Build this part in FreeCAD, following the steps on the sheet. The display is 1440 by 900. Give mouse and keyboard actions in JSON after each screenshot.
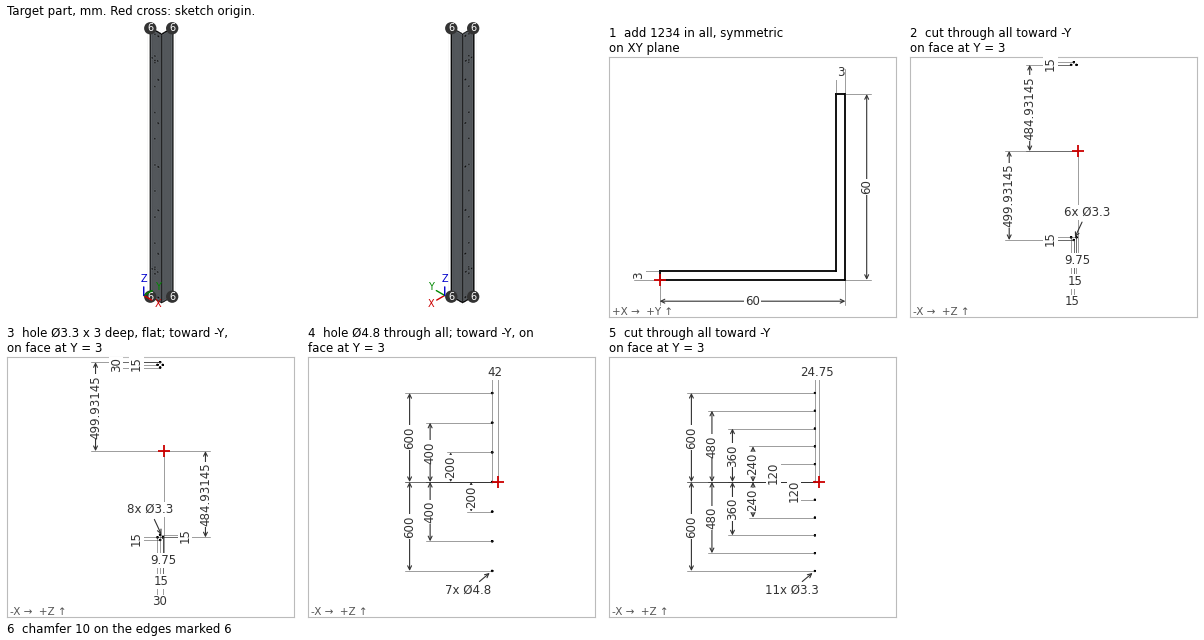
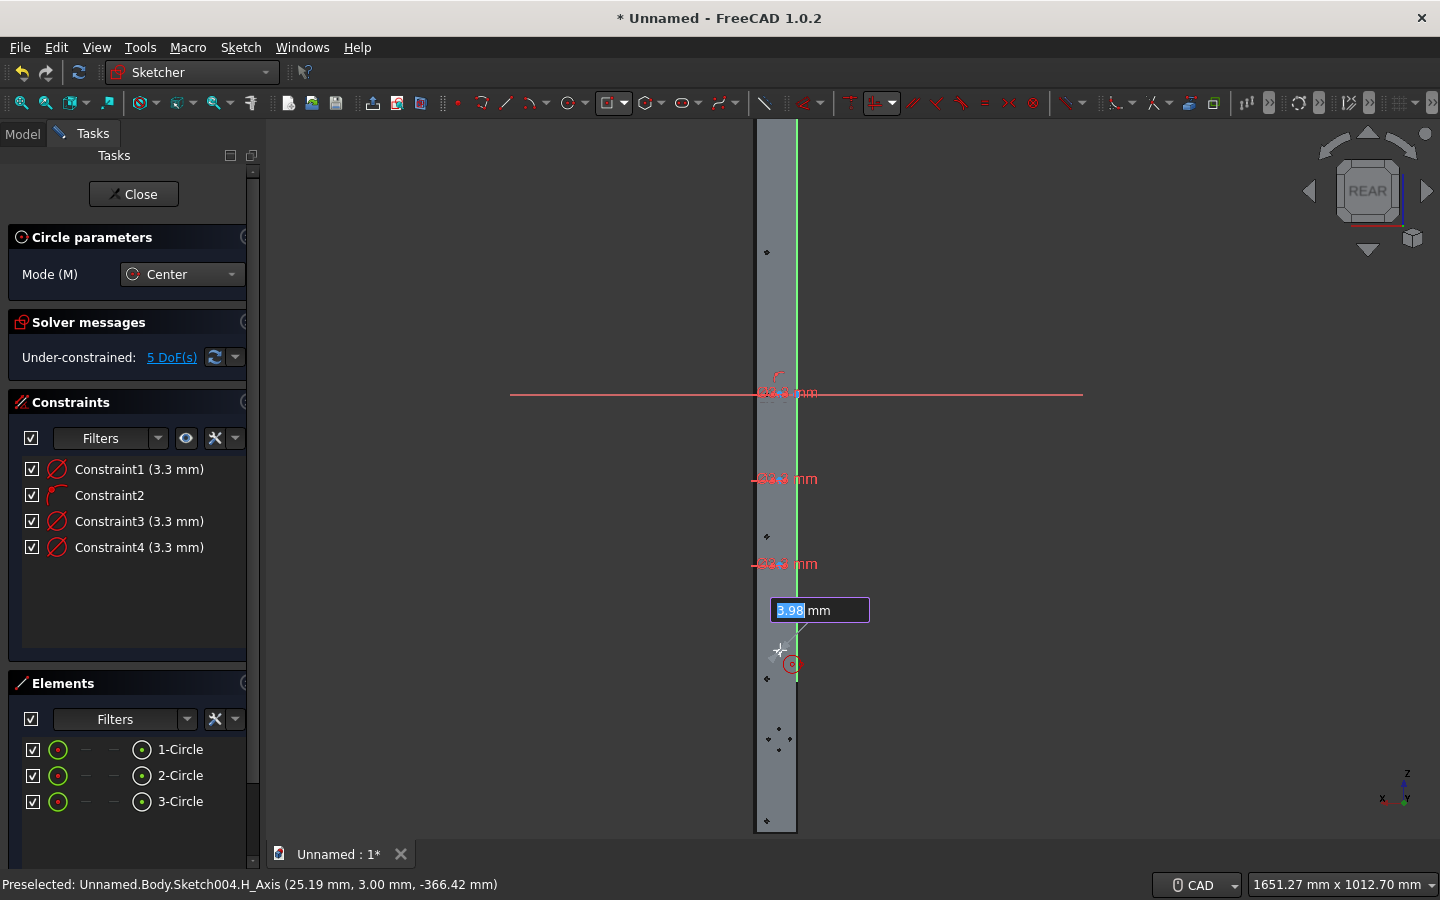
{"action": "type", "text": "3.3"}
{"action": "key", "text": "Return"}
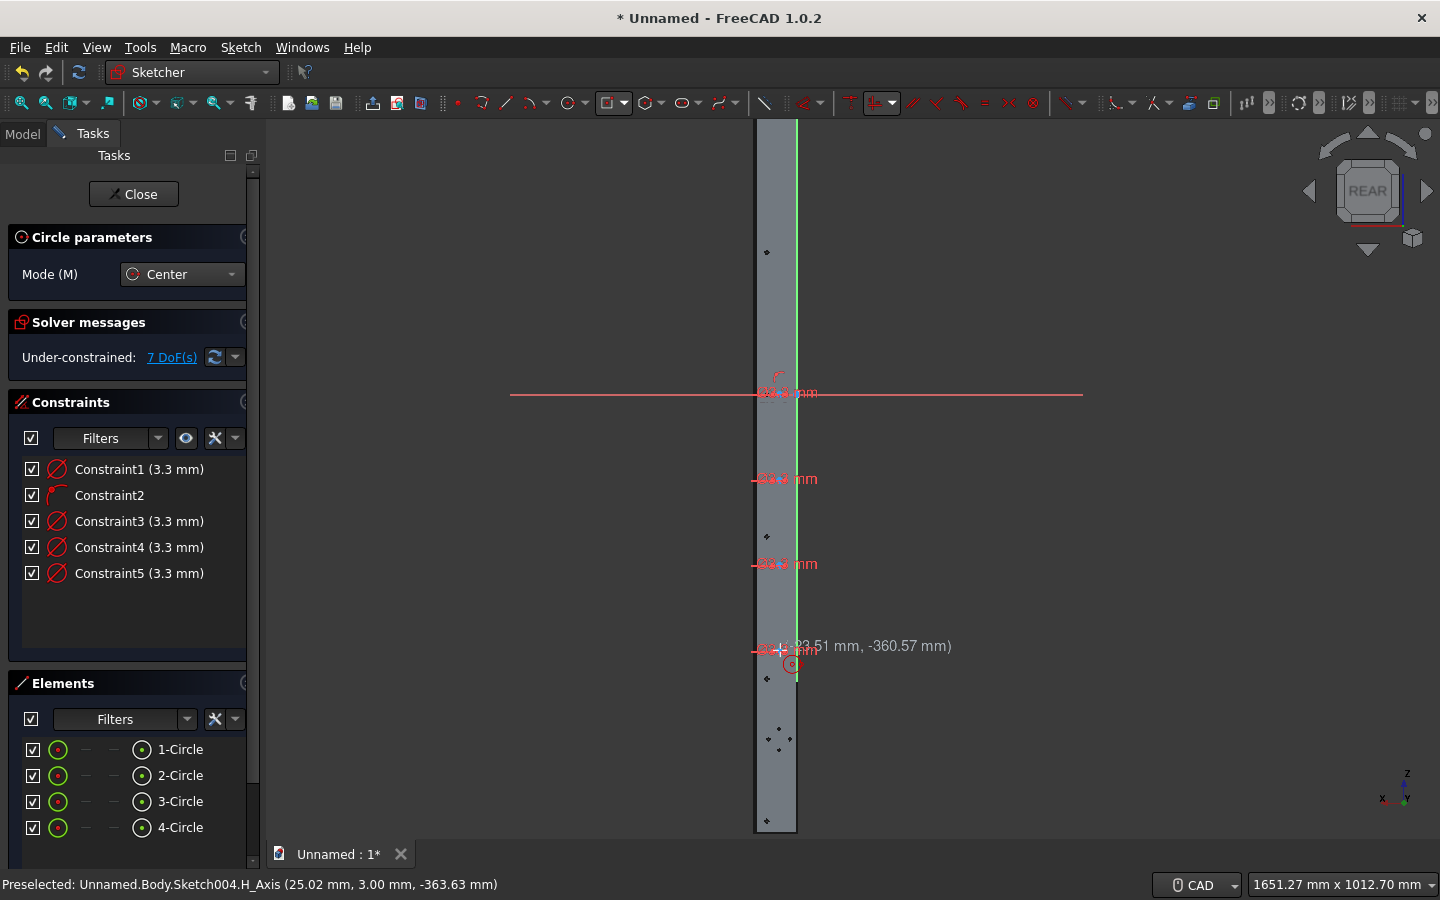
{"action": "scroll", "coordinate": [779, 736], "scroll_direction": "up", "scroll_amount": 15}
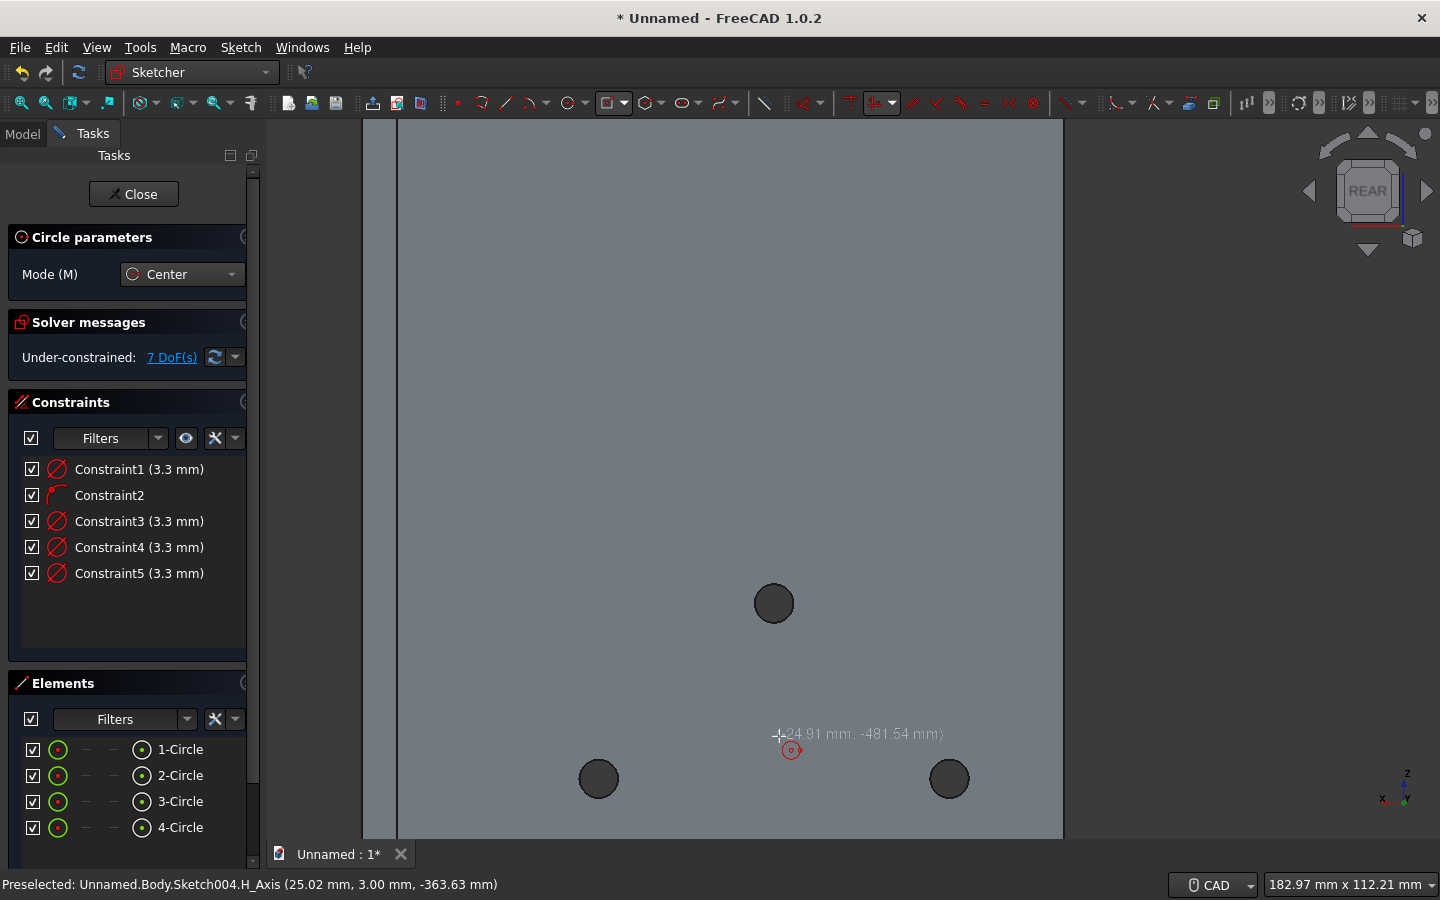
{"action": "scroll", "coordinate": [779, 707], "scroll_direction": "down", "scroll_amount": 17}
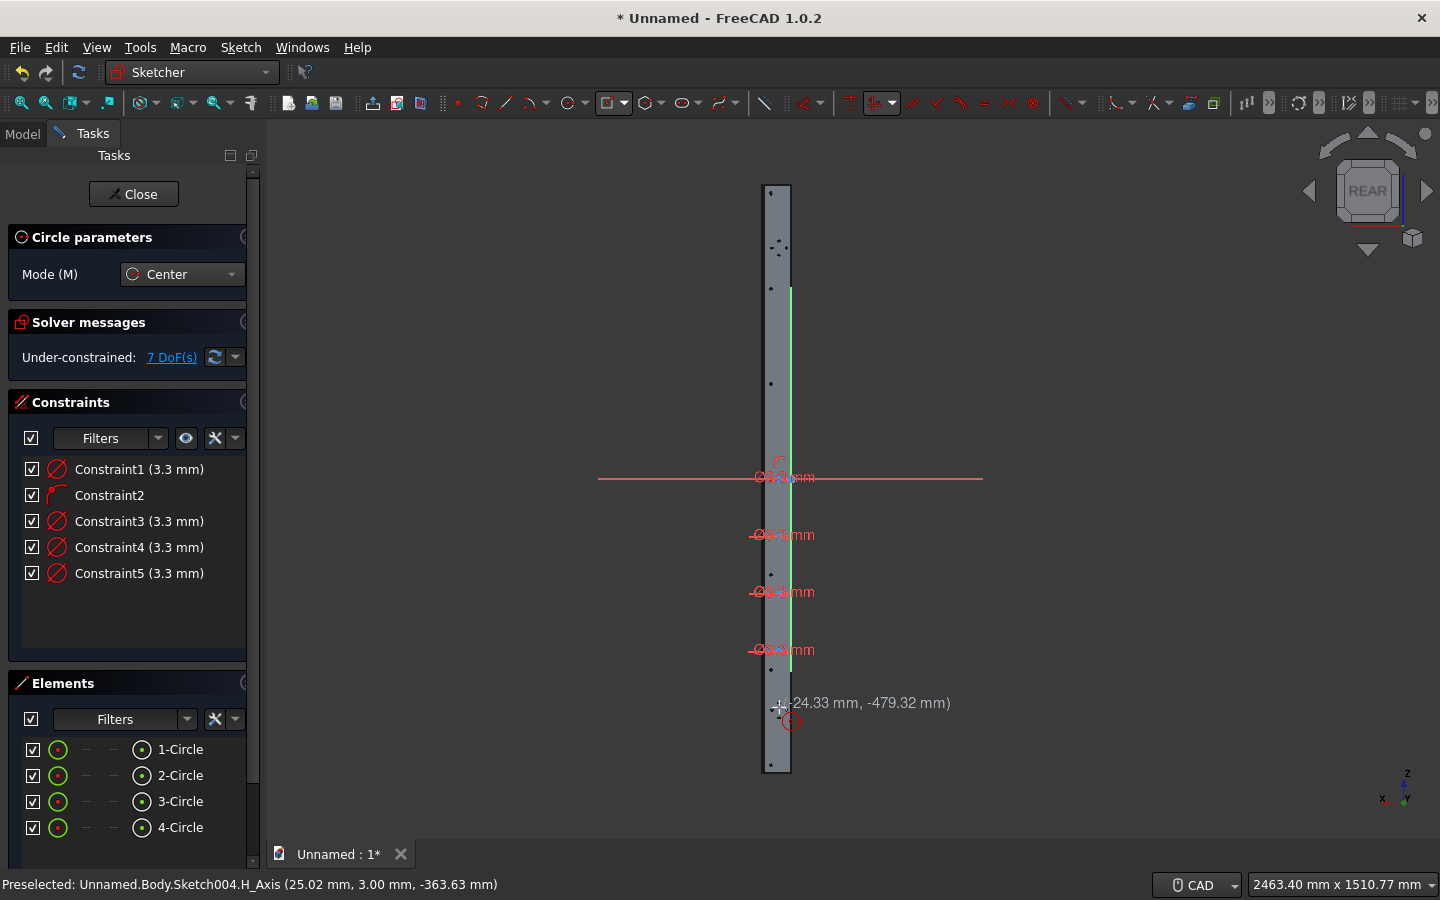
{"action": "scroll", "coordinate": [779, 708], "scroll_direction": "up", "scroll_amount": 2}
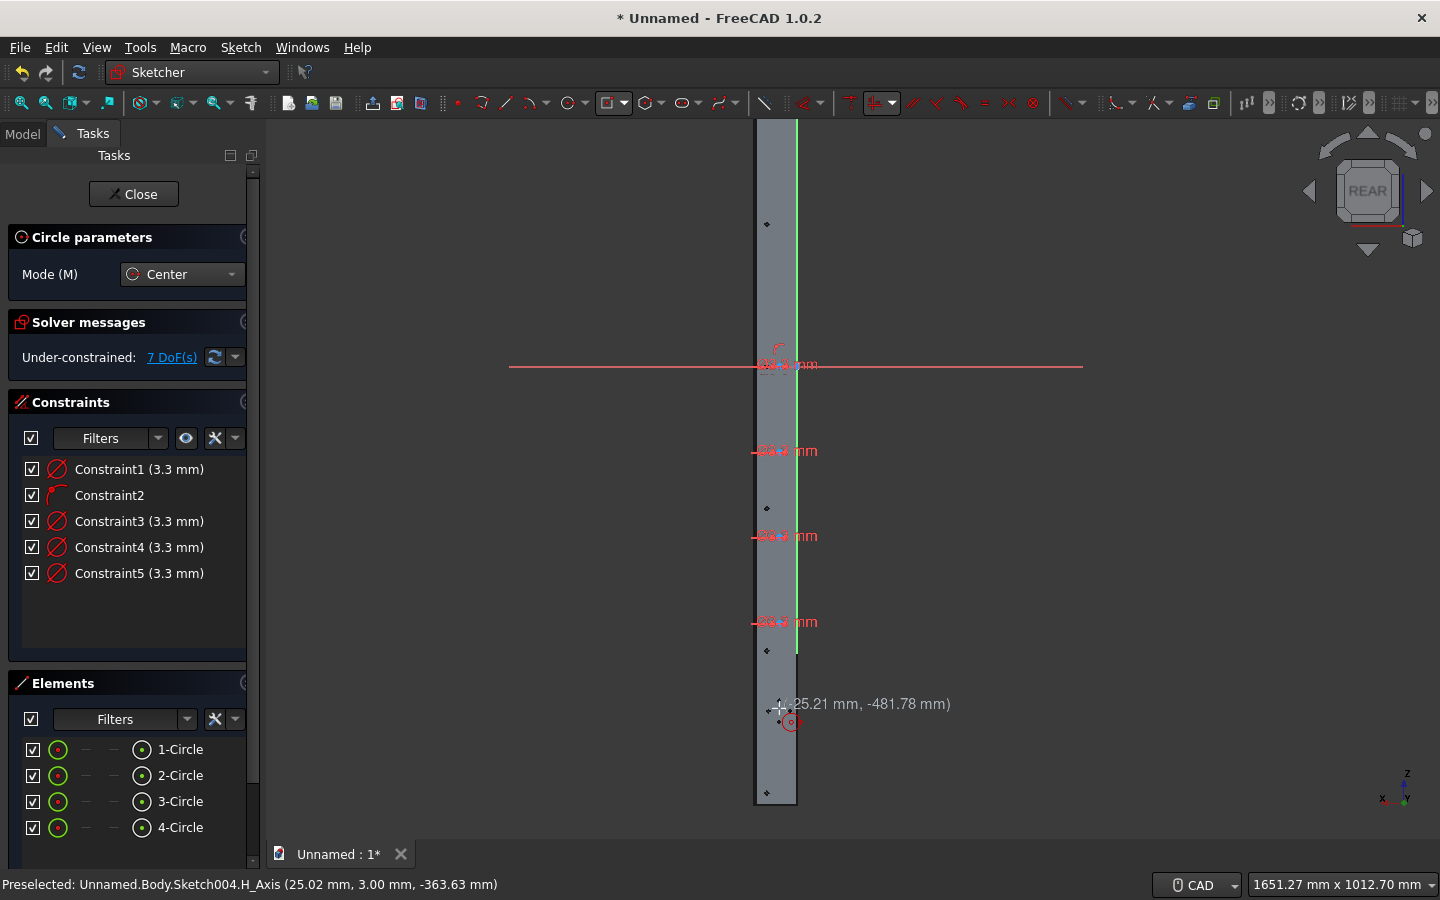
{"action": "left_click", "coordinate": [779, 708]}
{"action": "mouse_move", "coordinate": [780, 707]}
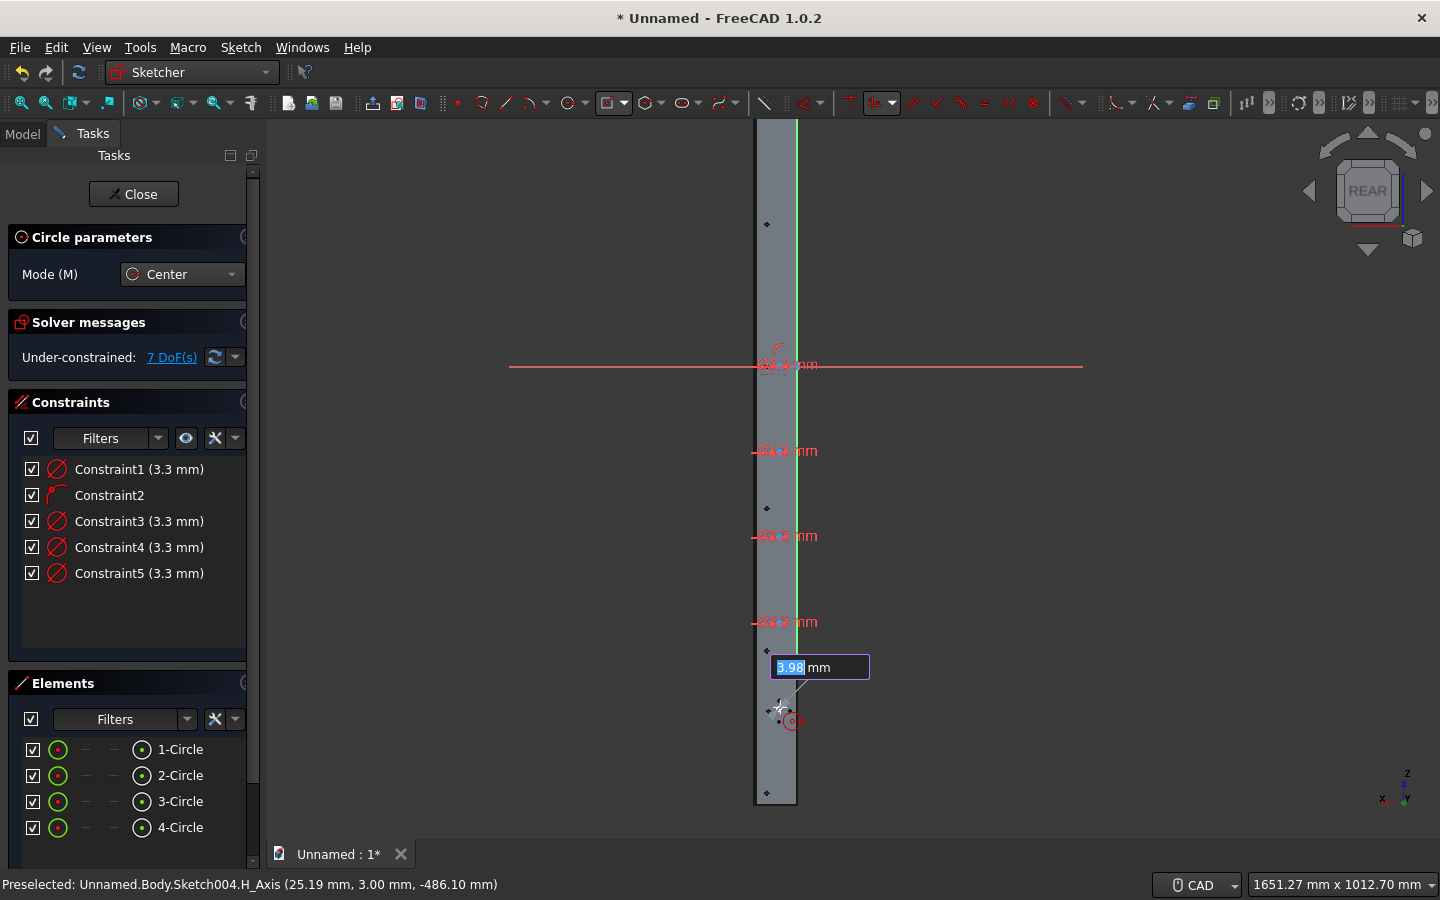
{"action": "type", "text": "3.3"}
{"action": "key", "text": "Return"}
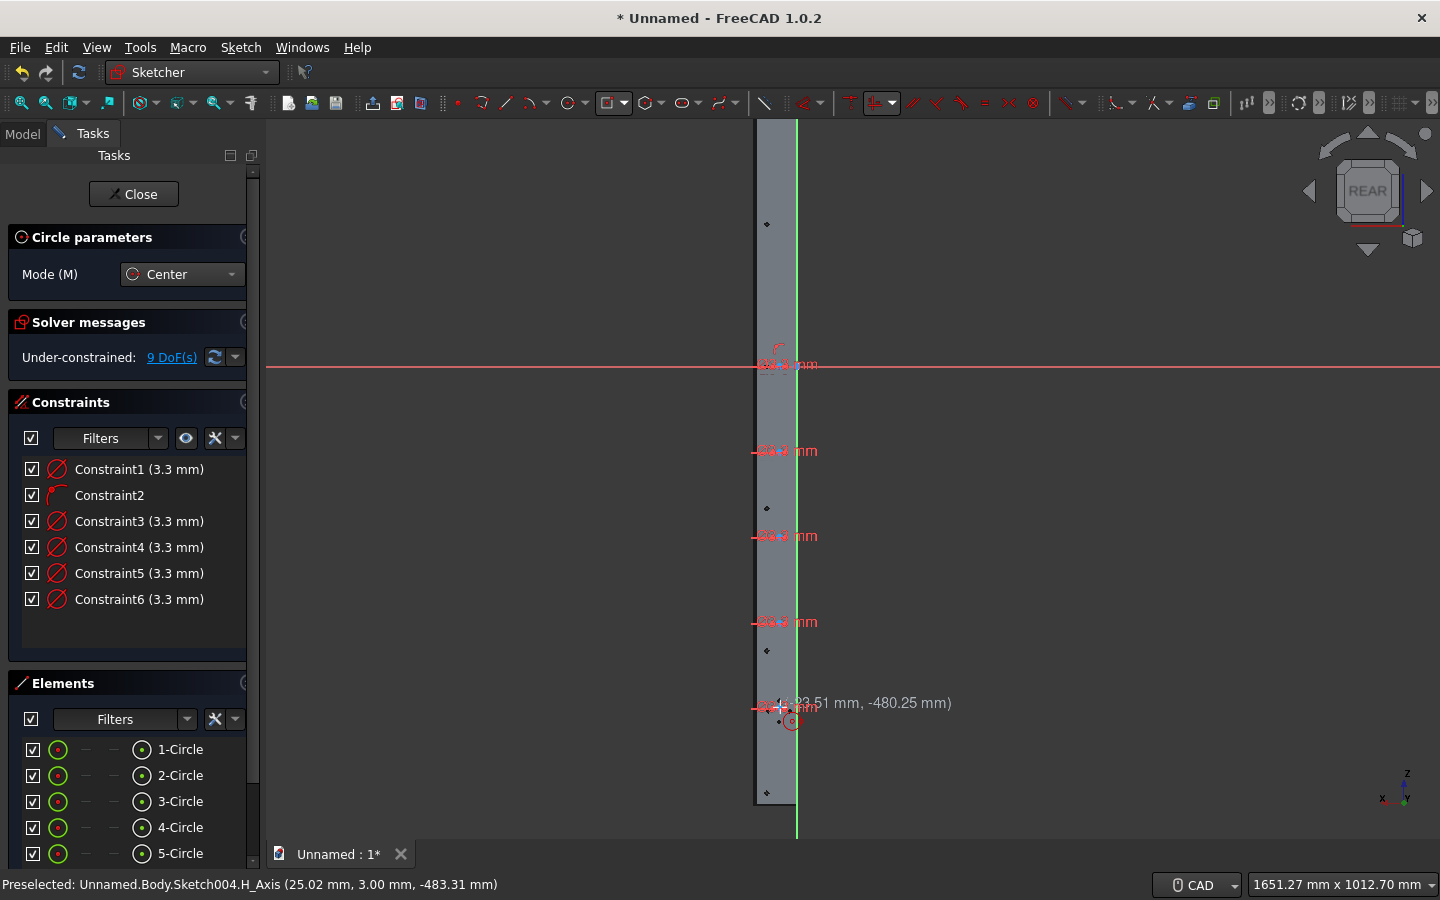
{"action": "scroll", "coordinate": [779, 793], "scroll_direction": "up", "scroll_amount": 15}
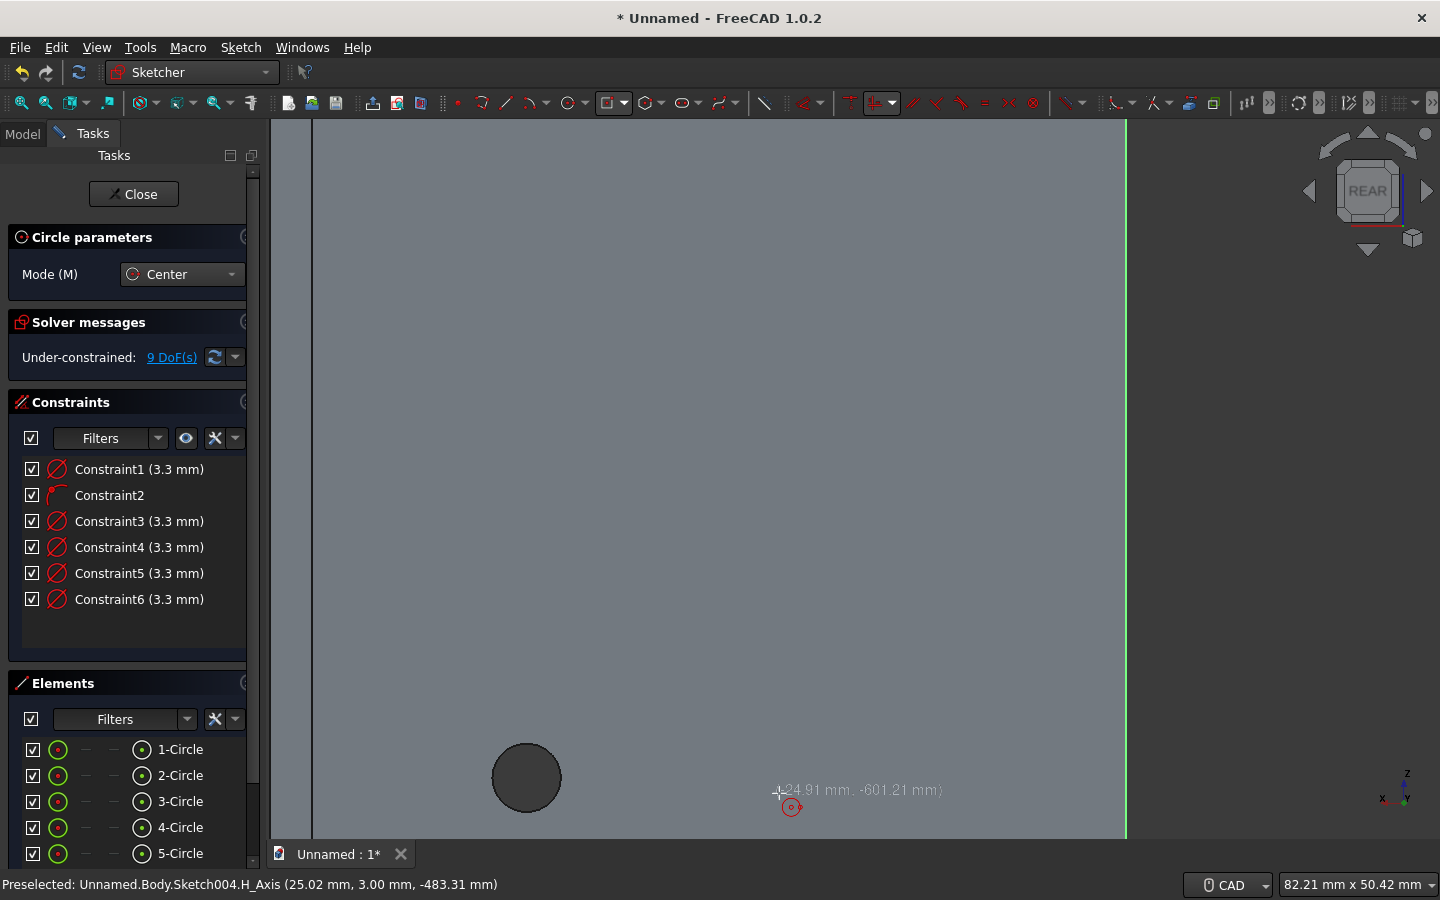
{"action": "scroll", "coordinate": [779, 765], "scroll_direction": "down", "scroll_amount": 17}